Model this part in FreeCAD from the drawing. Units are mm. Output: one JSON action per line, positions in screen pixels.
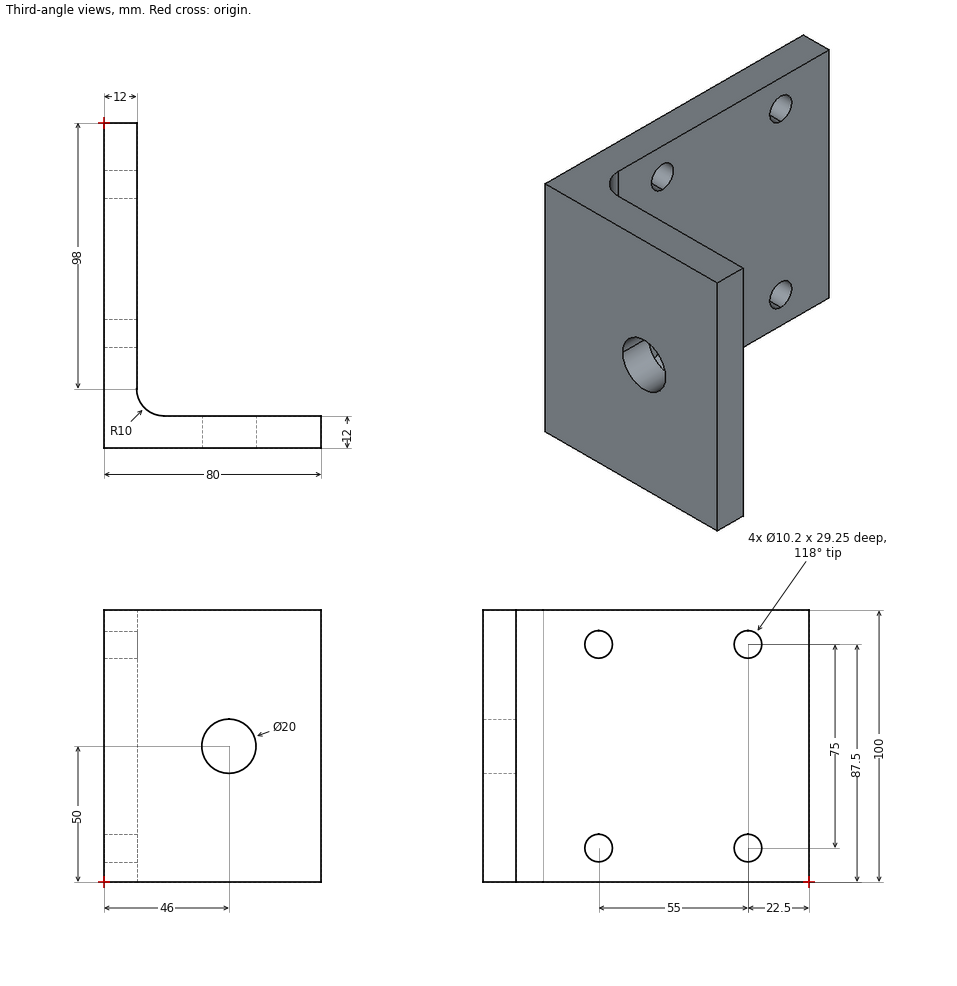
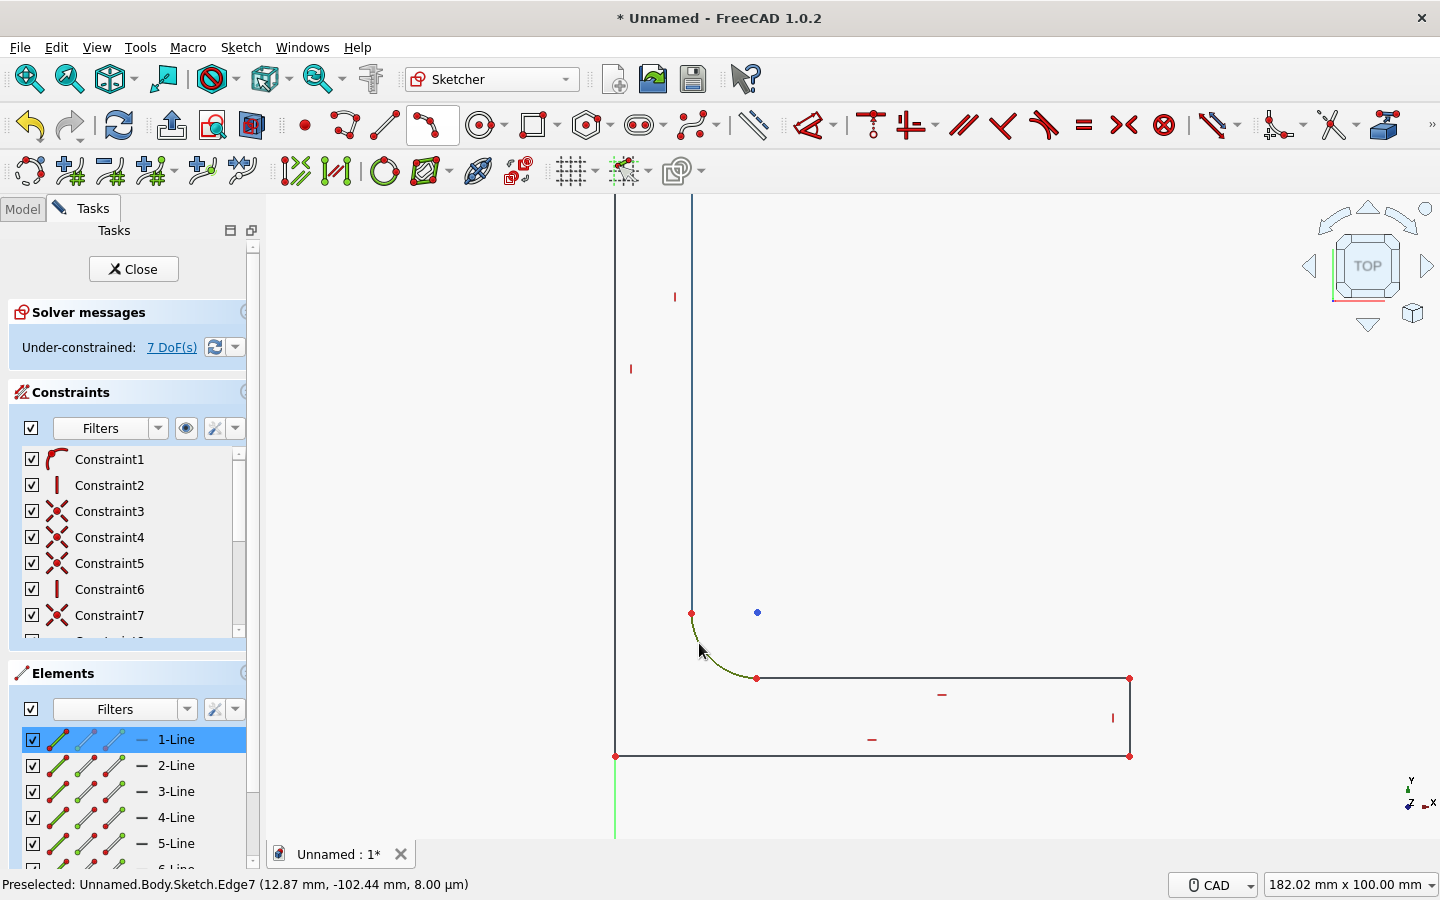
{"action": "left_click", "coordinate": [1044, 126]}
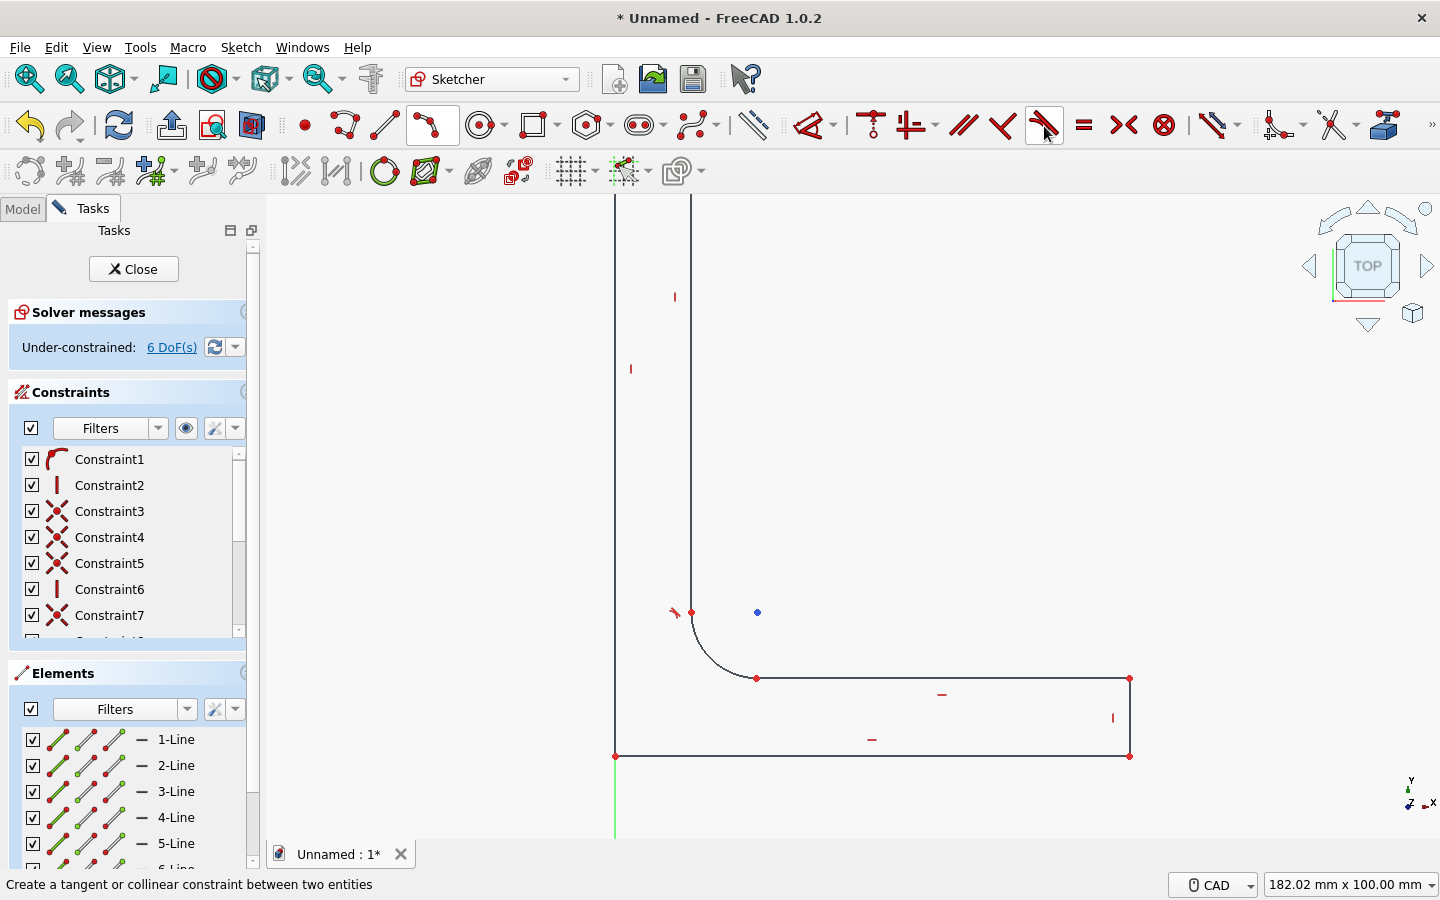
{"action": "left_click", "coordinate": [1018, 678]}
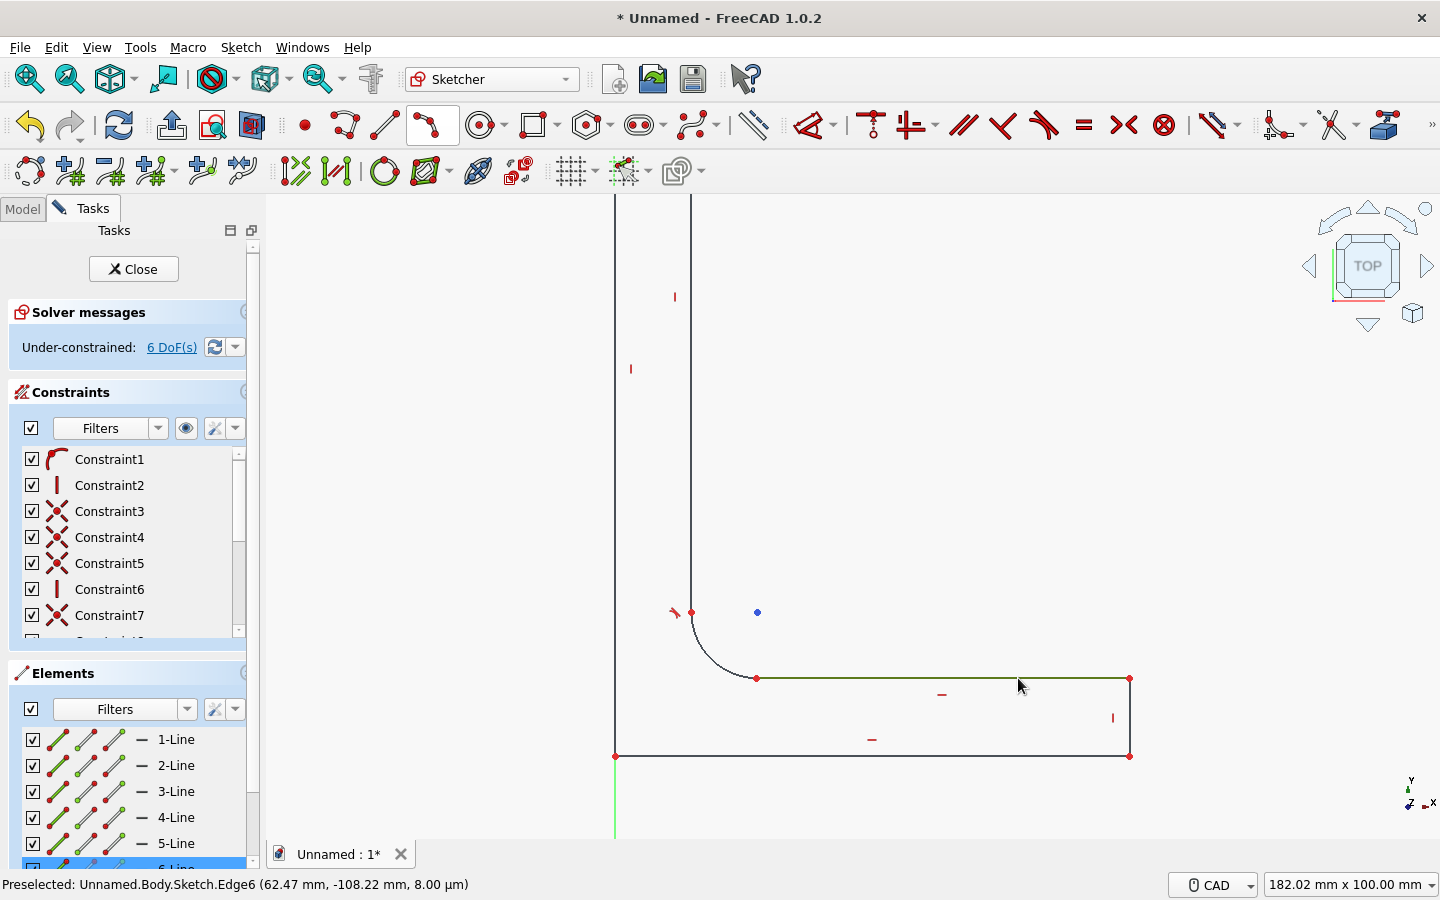
{"action": "left_click", "coordinate": [698, 642]}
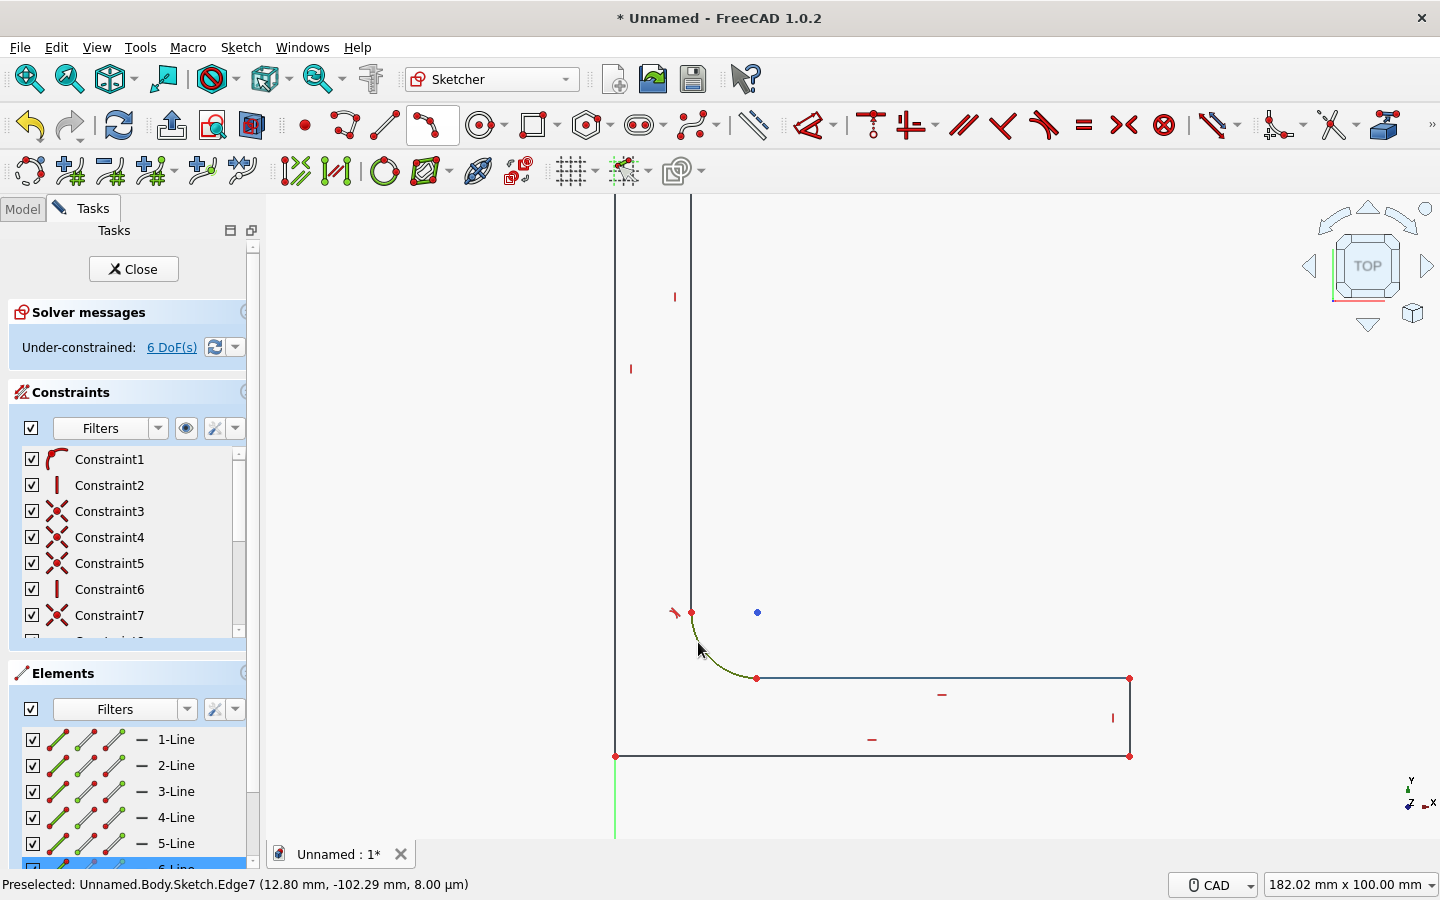
{"action": "left_click", "coordinate": [1044, 126]}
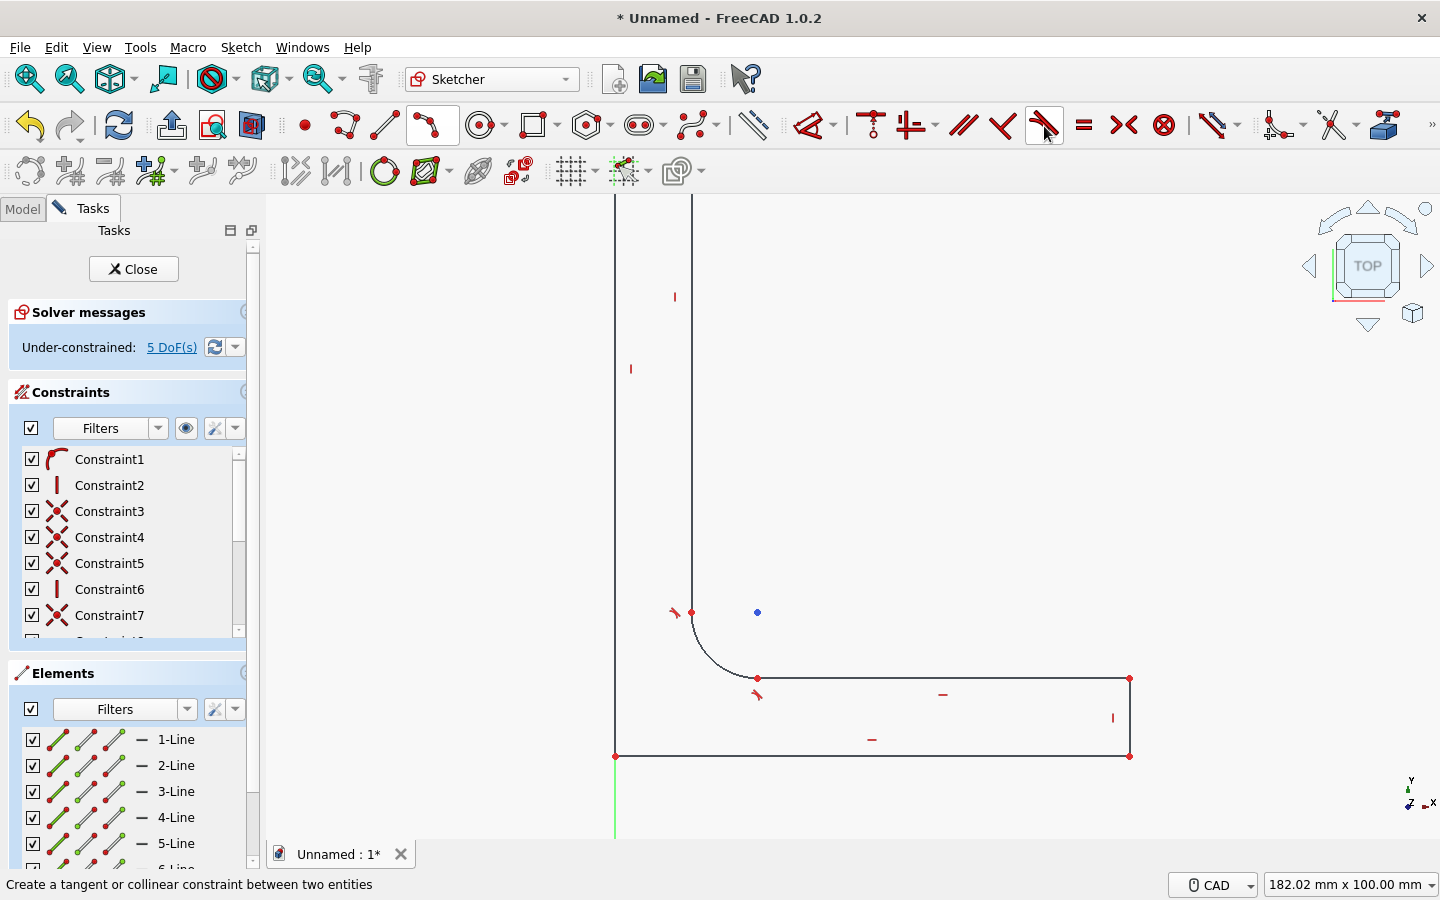
{"action": "left_click", "coordinate": [808, 126]}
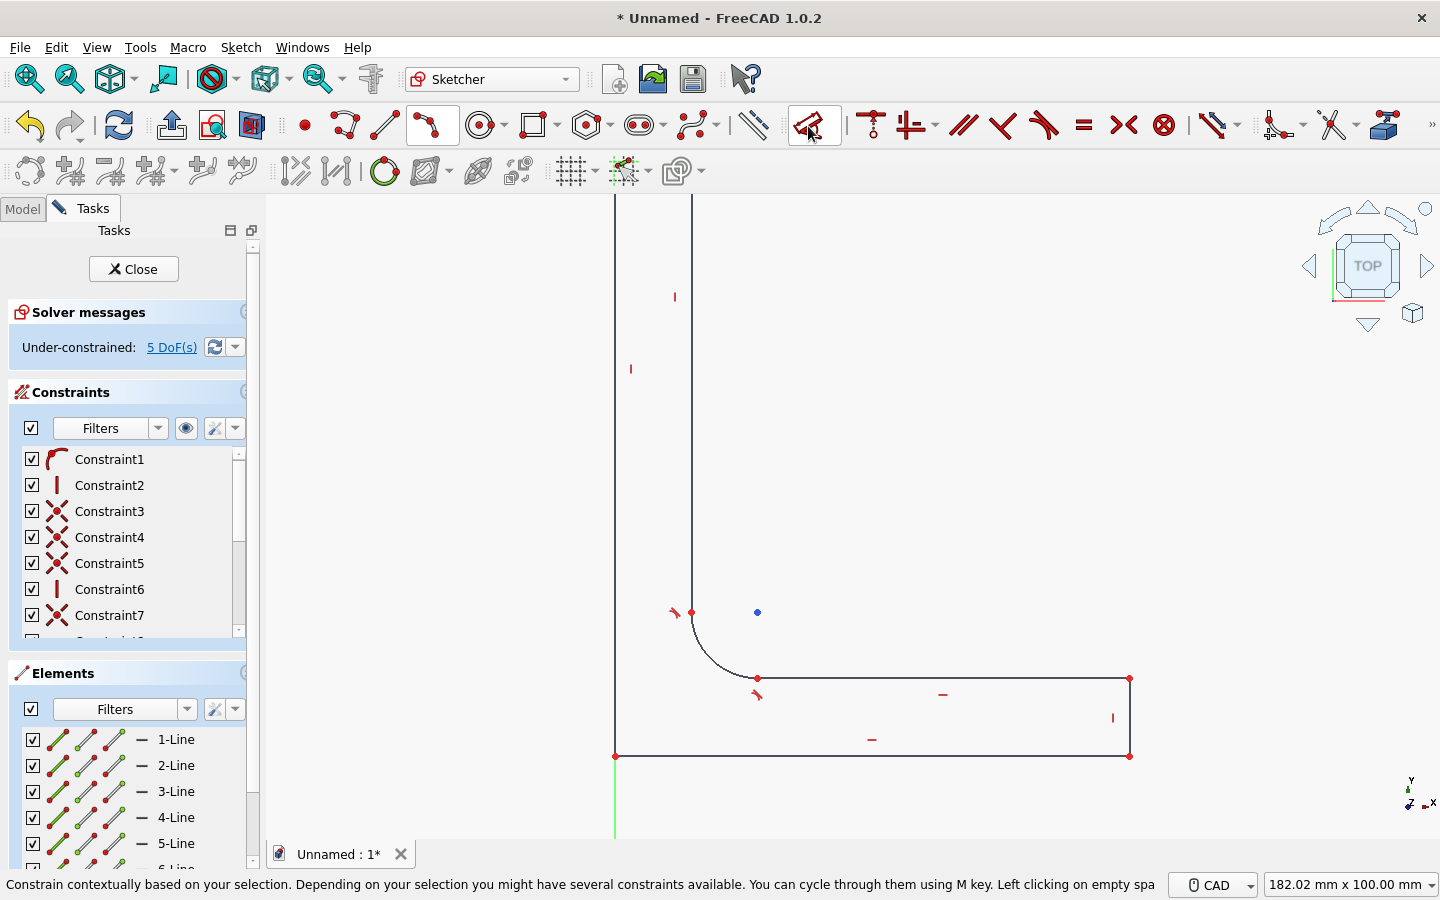
{"action": "left_click", "coordinate": [699, 642]}
{"action": "left_click", "coordinate": [670, 657]}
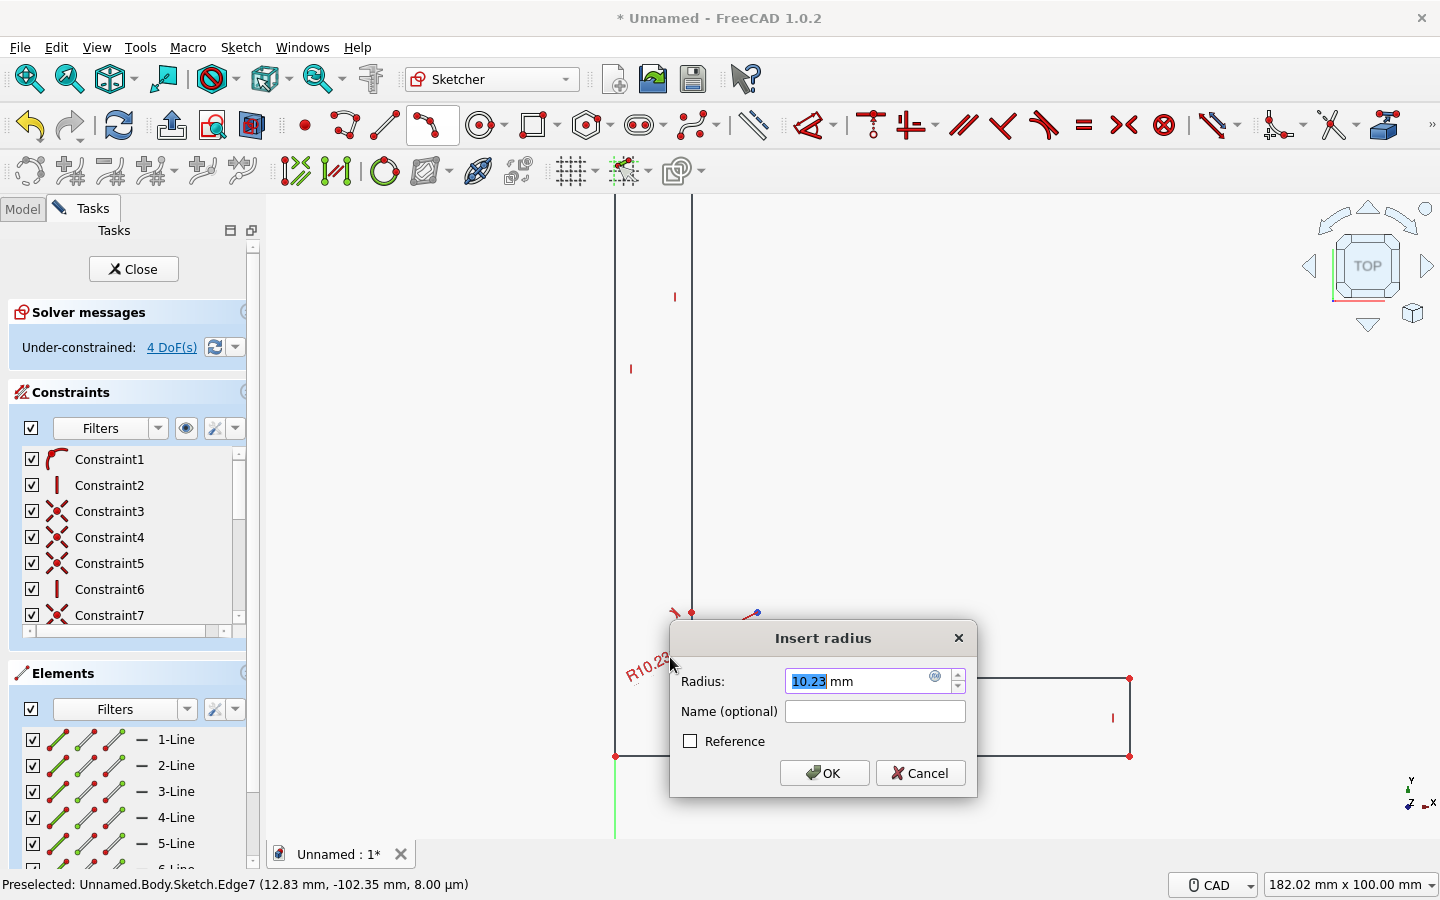
{"action": "type", "text": "10"}
{"action": "key", "text": "Return"}